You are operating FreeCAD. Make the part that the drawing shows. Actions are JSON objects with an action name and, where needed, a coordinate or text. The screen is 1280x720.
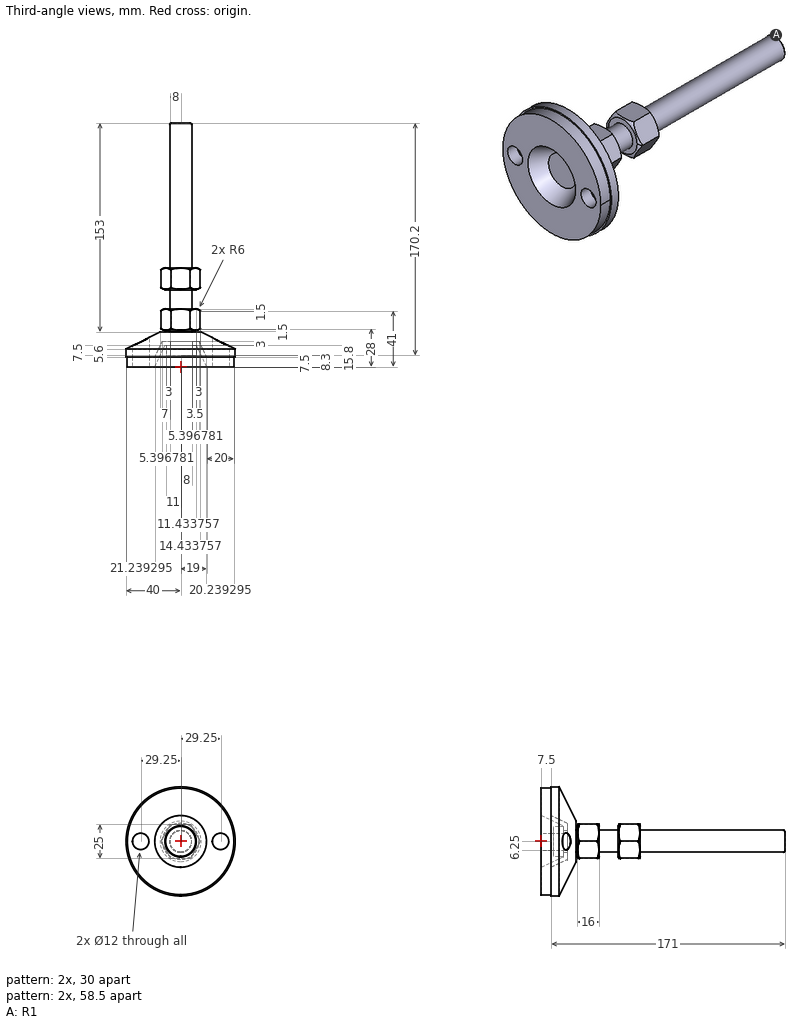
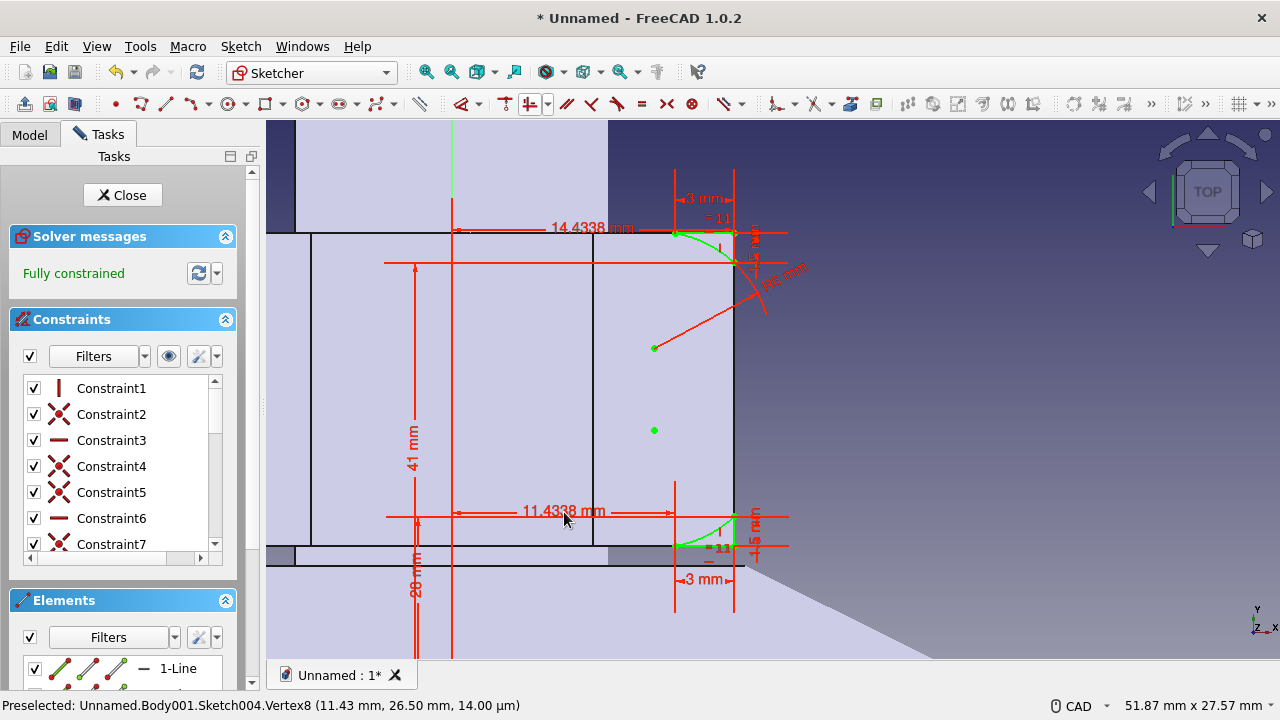
{"action": "left_click", "coordinate": [123, 195]}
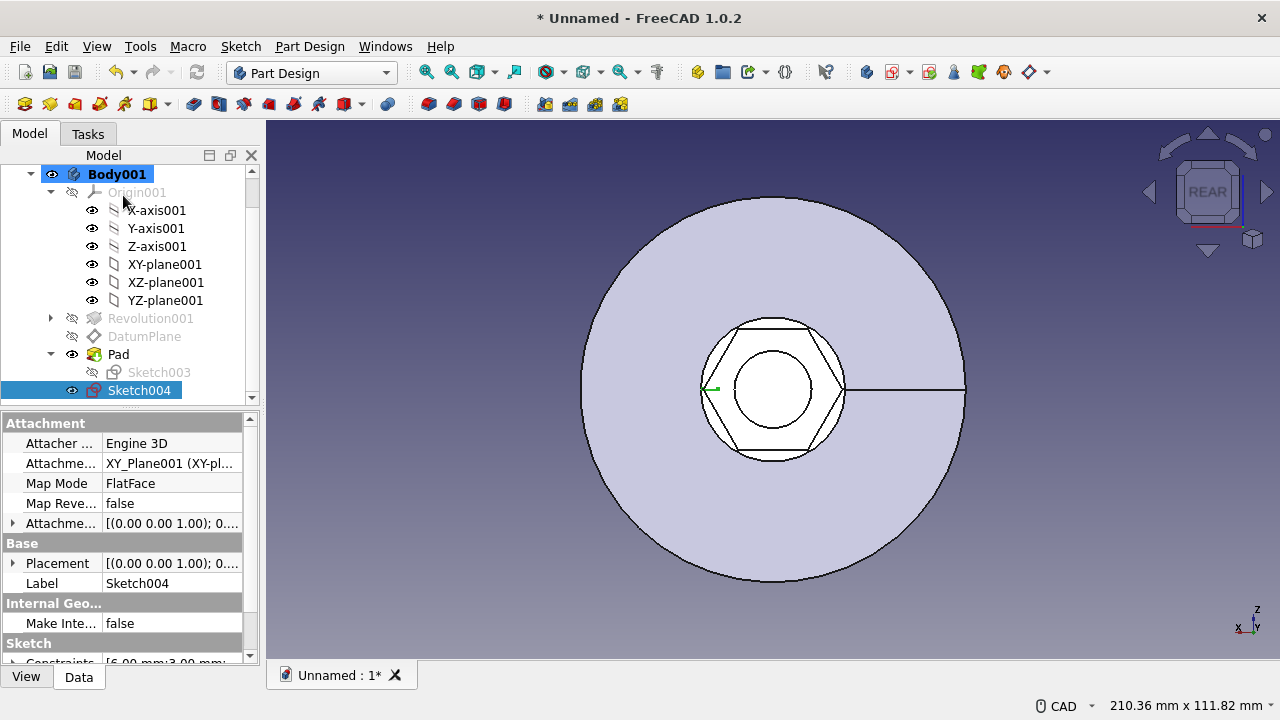
{"action": "left_click", "coordinate": [244, 104]}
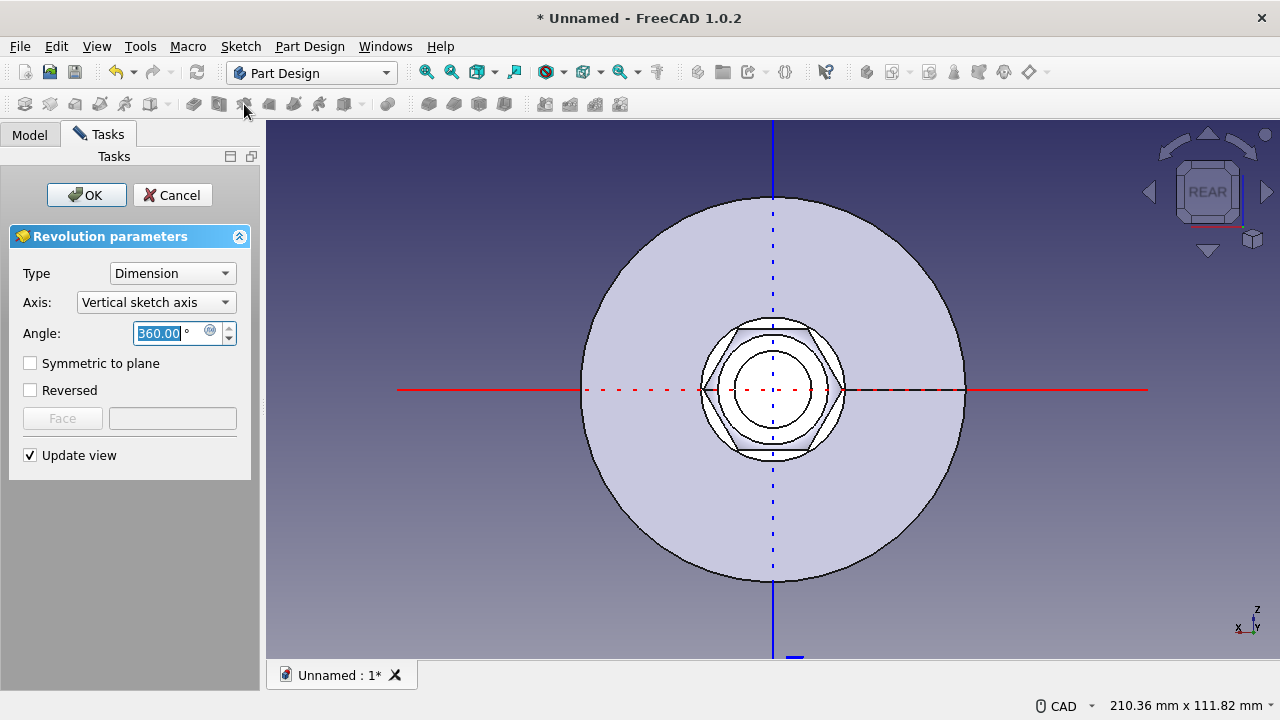
{"action": "left_click", "coordinate": [87, 195]}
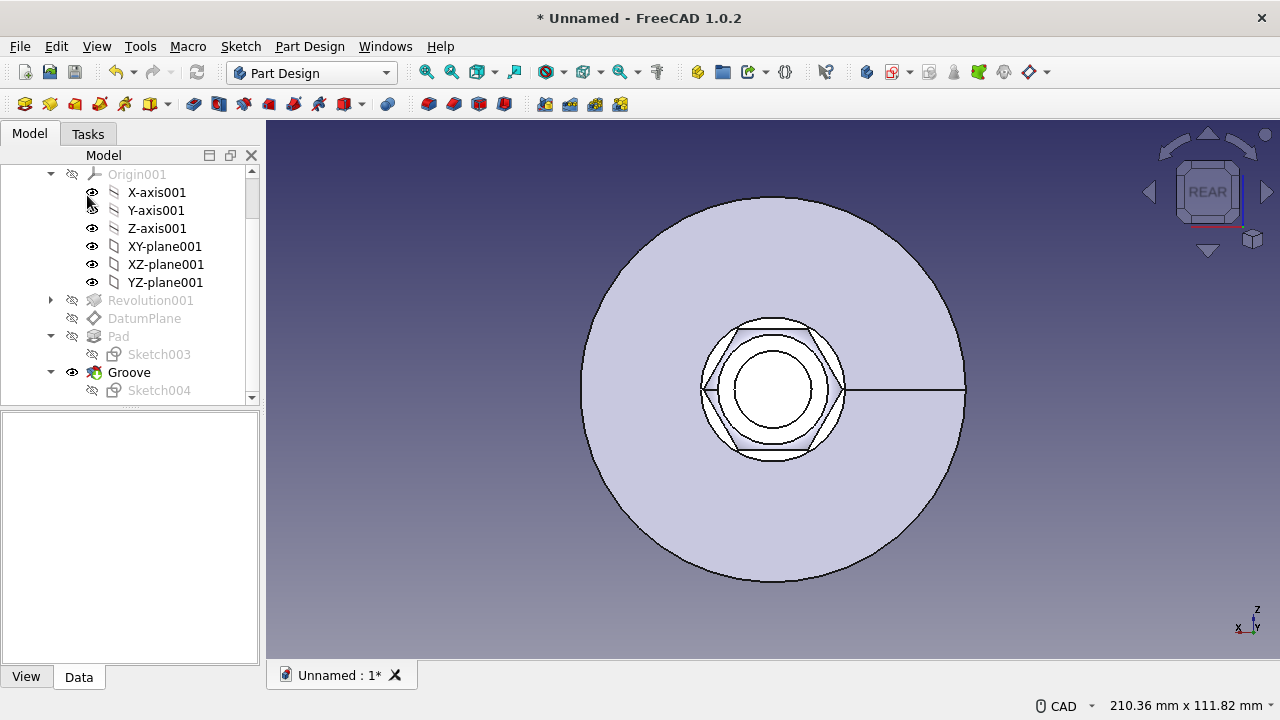
{"action": "left_click", "coordinate": [117, 336]}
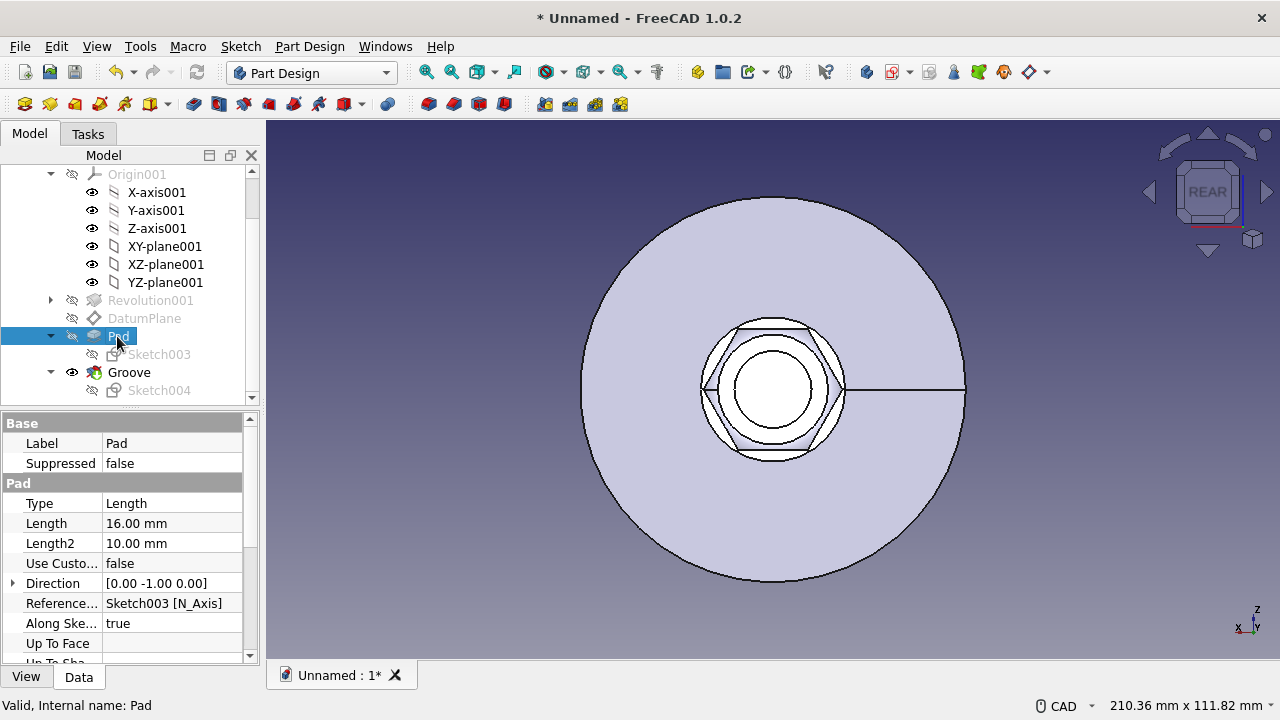
{"action": "left_click", "coordinate": [117, 372], "text": "ctrl"}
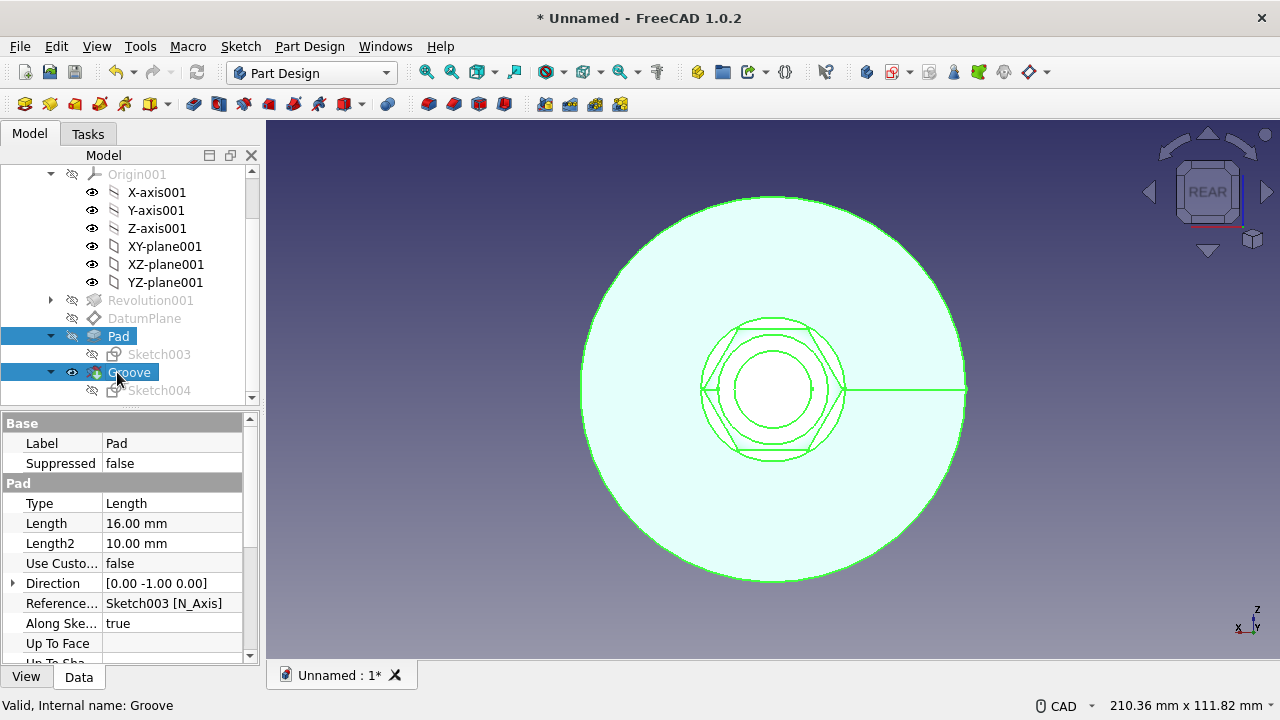
{"action": "left_click", "coordinate": [570, 104]}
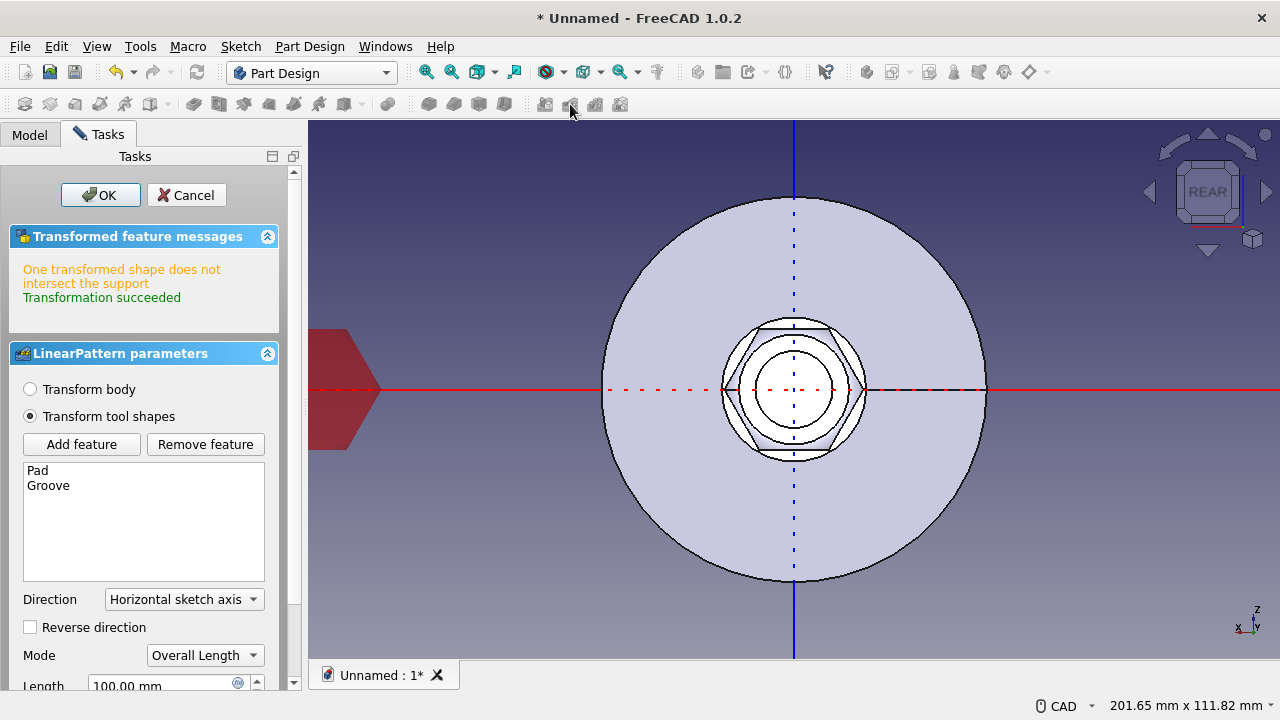
{"action": "left_click", "coordinate": [185, 600]}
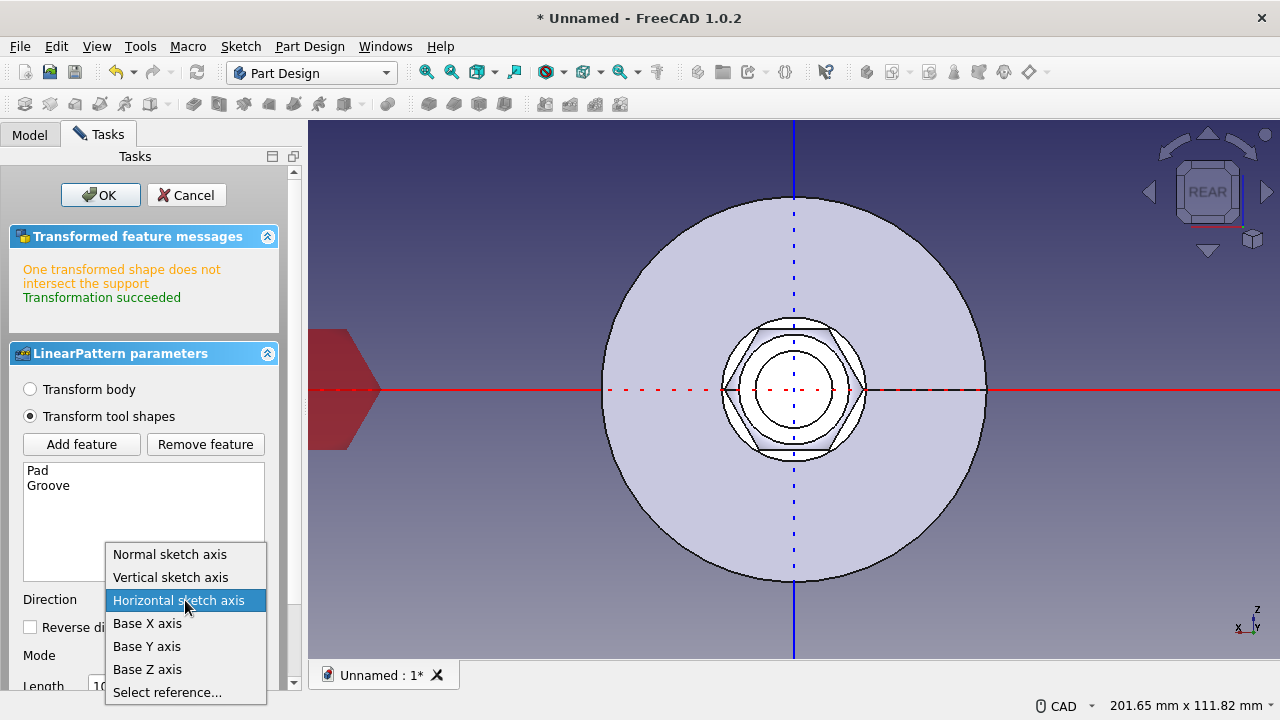
{"action": "left_click", "coordinate": [184, 646]}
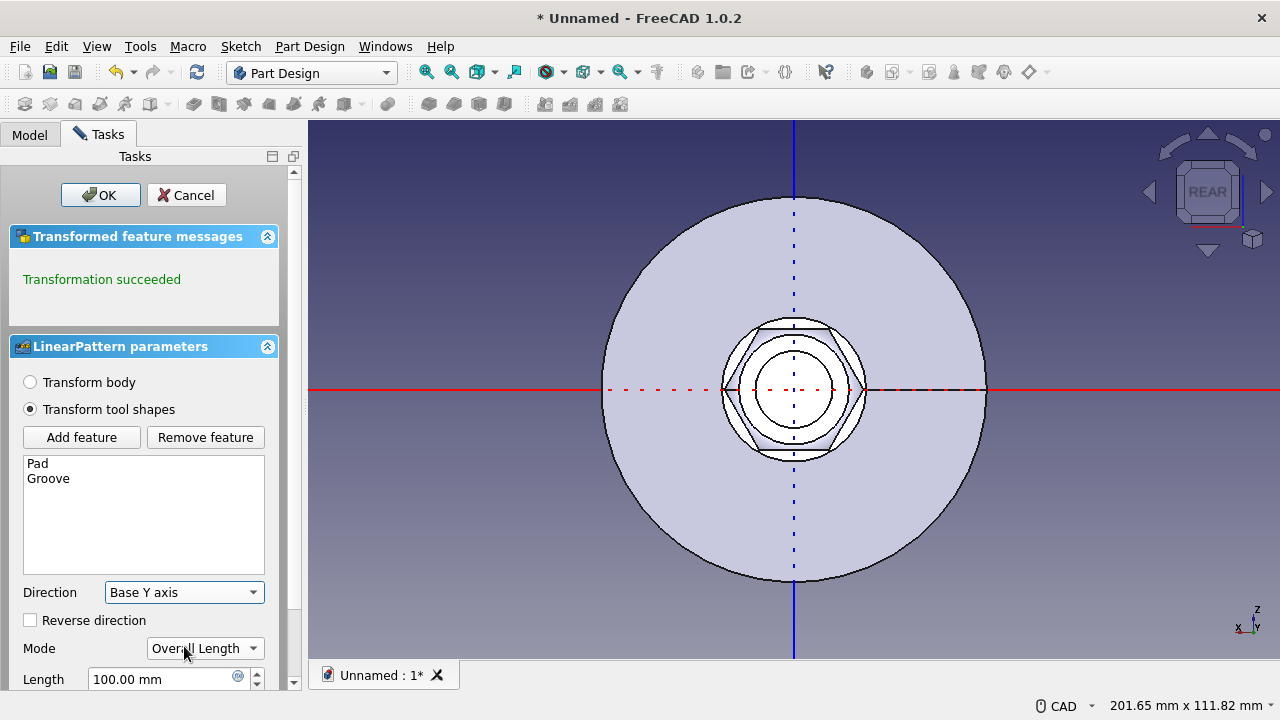
{"action": "left_click", "coordinate": [206, 648]}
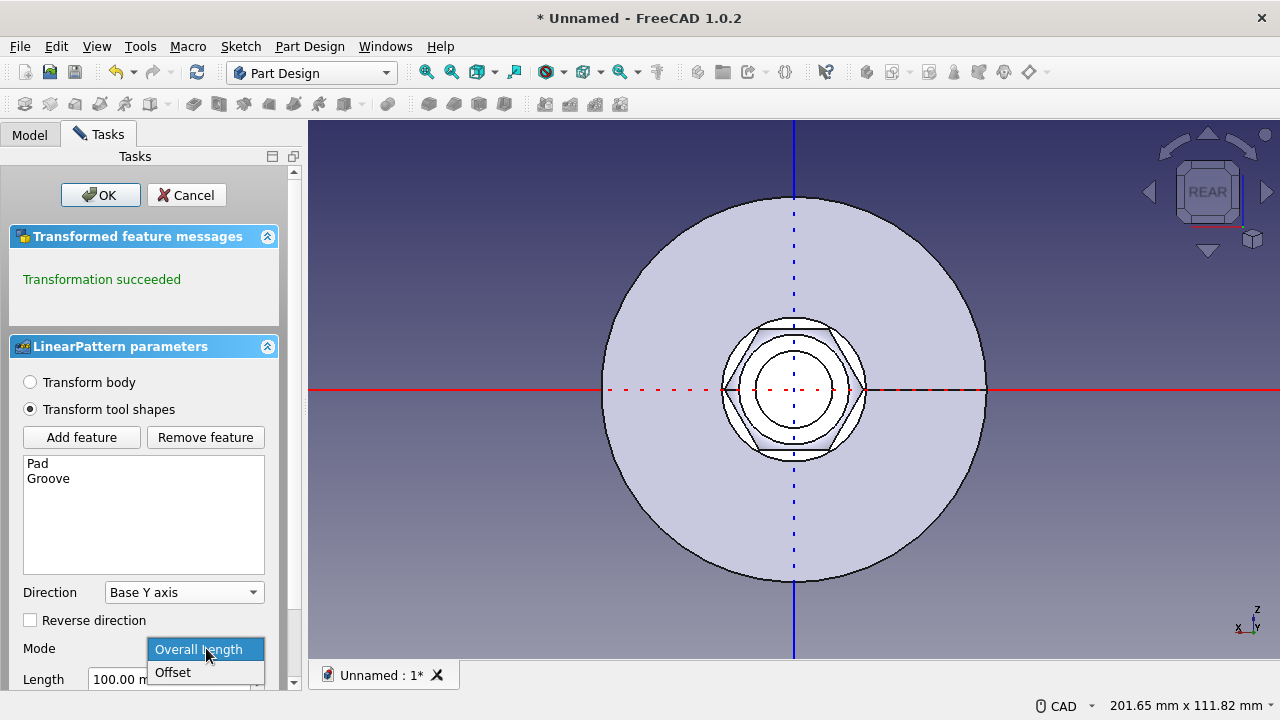
{"action": "left_click", "coordinate": [204, 672]}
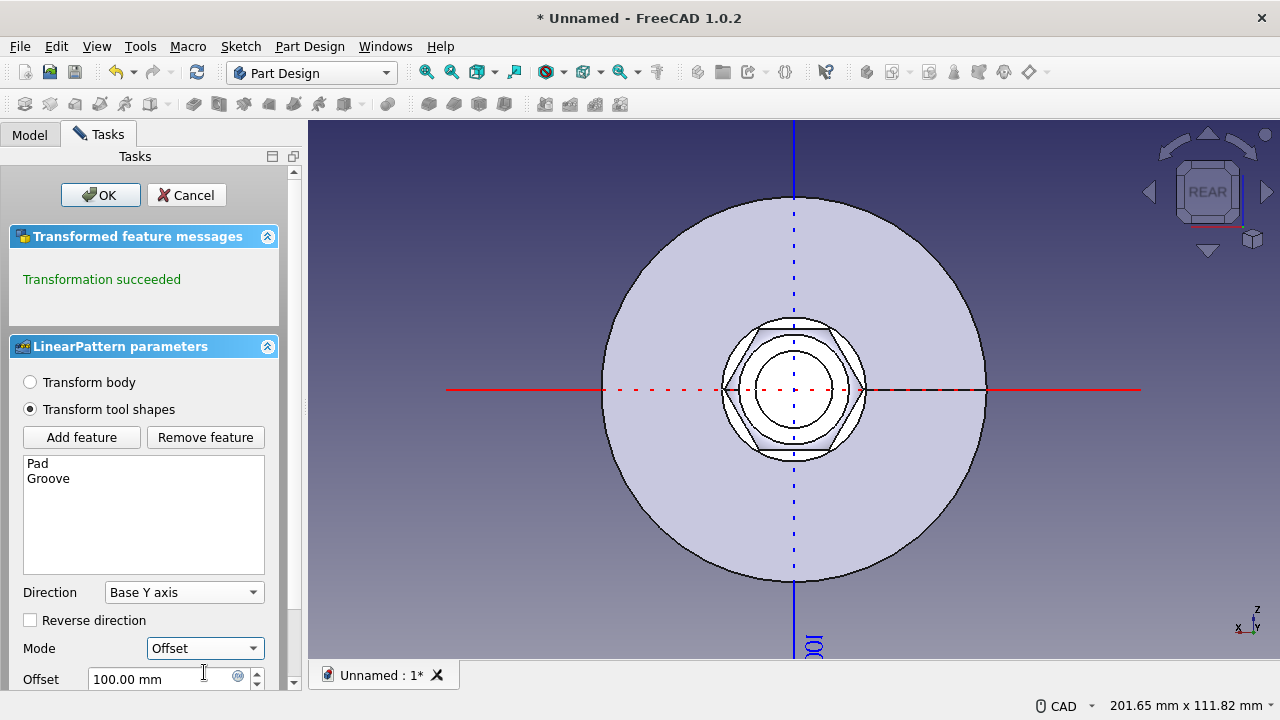
{"action": "scroll", "coordinate": [294, 428], "scroll_direction": "down", "scroll_amount": 2}